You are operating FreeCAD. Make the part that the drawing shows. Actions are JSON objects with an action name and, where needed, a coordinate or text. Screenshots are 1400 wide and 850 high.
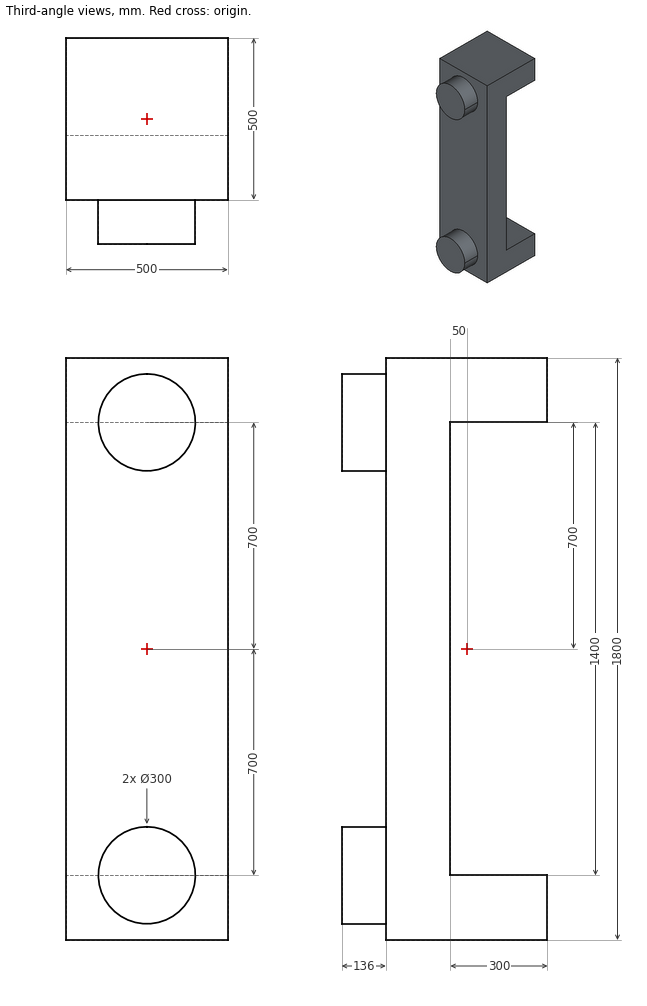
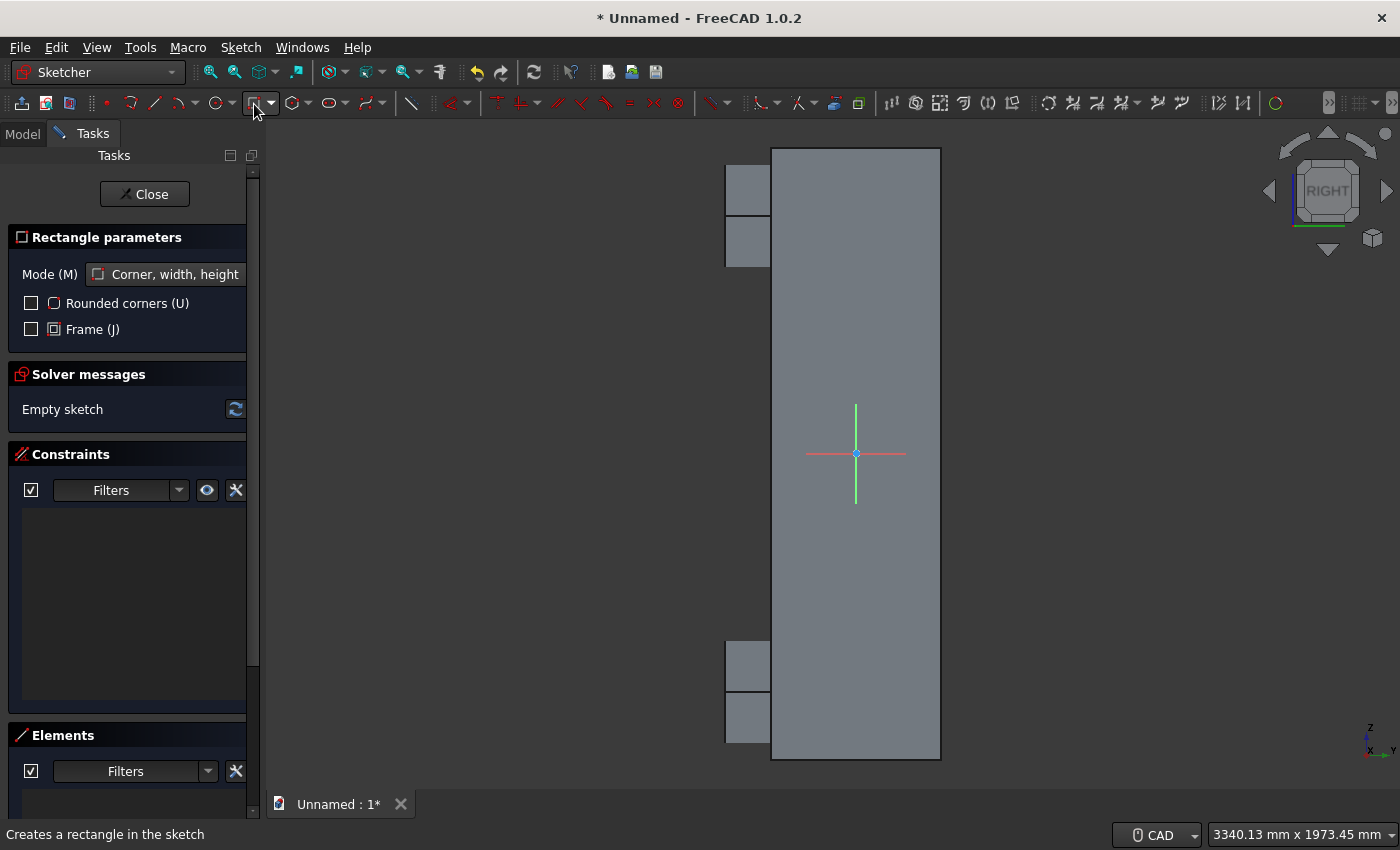
{"action": "left_click", "coordinate": [839, 216]}
{"action": "left_click", "coordinate": [941, 692]}
{"action": "key", "text": "Escape"}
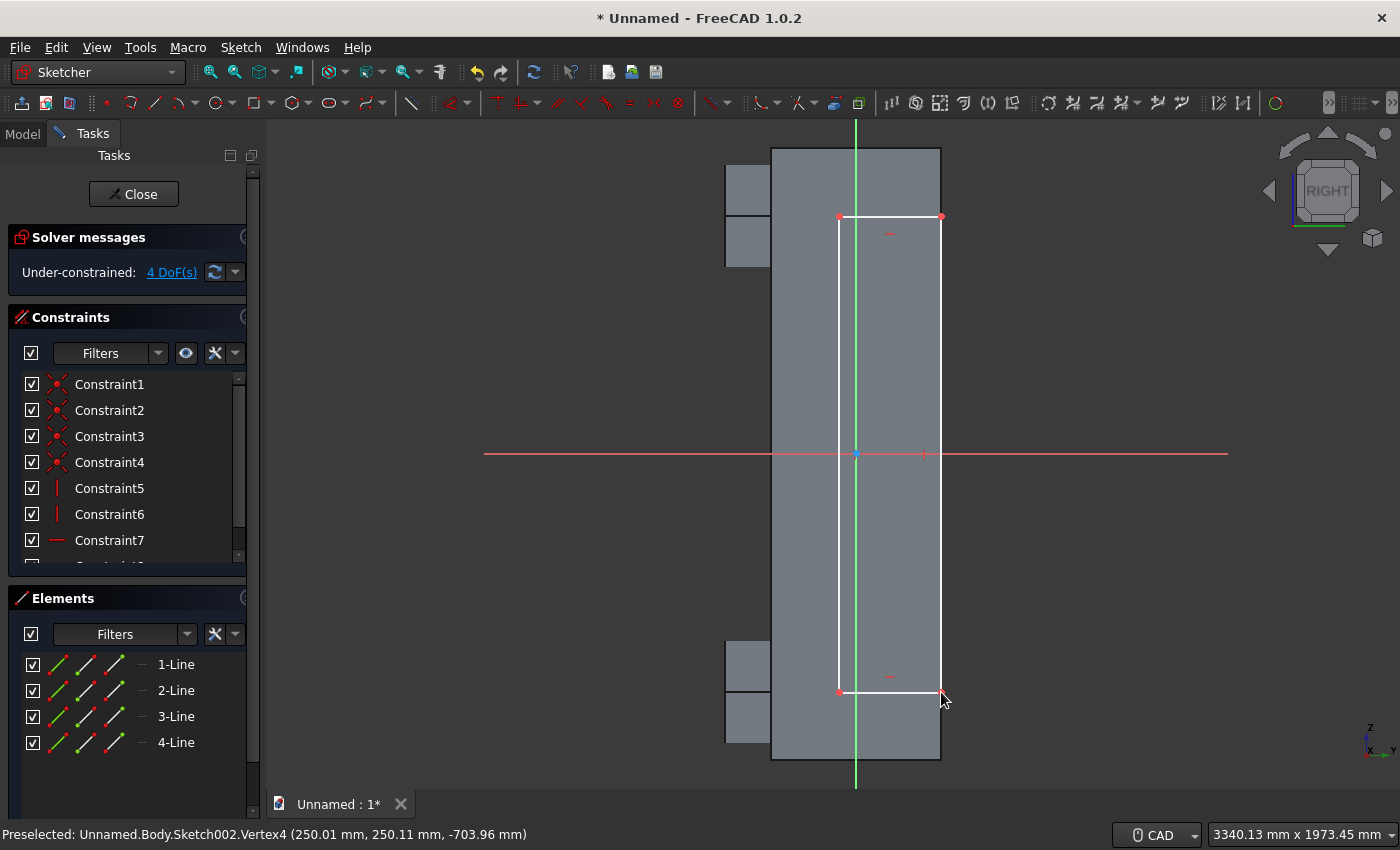
{"action": "left_click", "coordinate": [450, 104]}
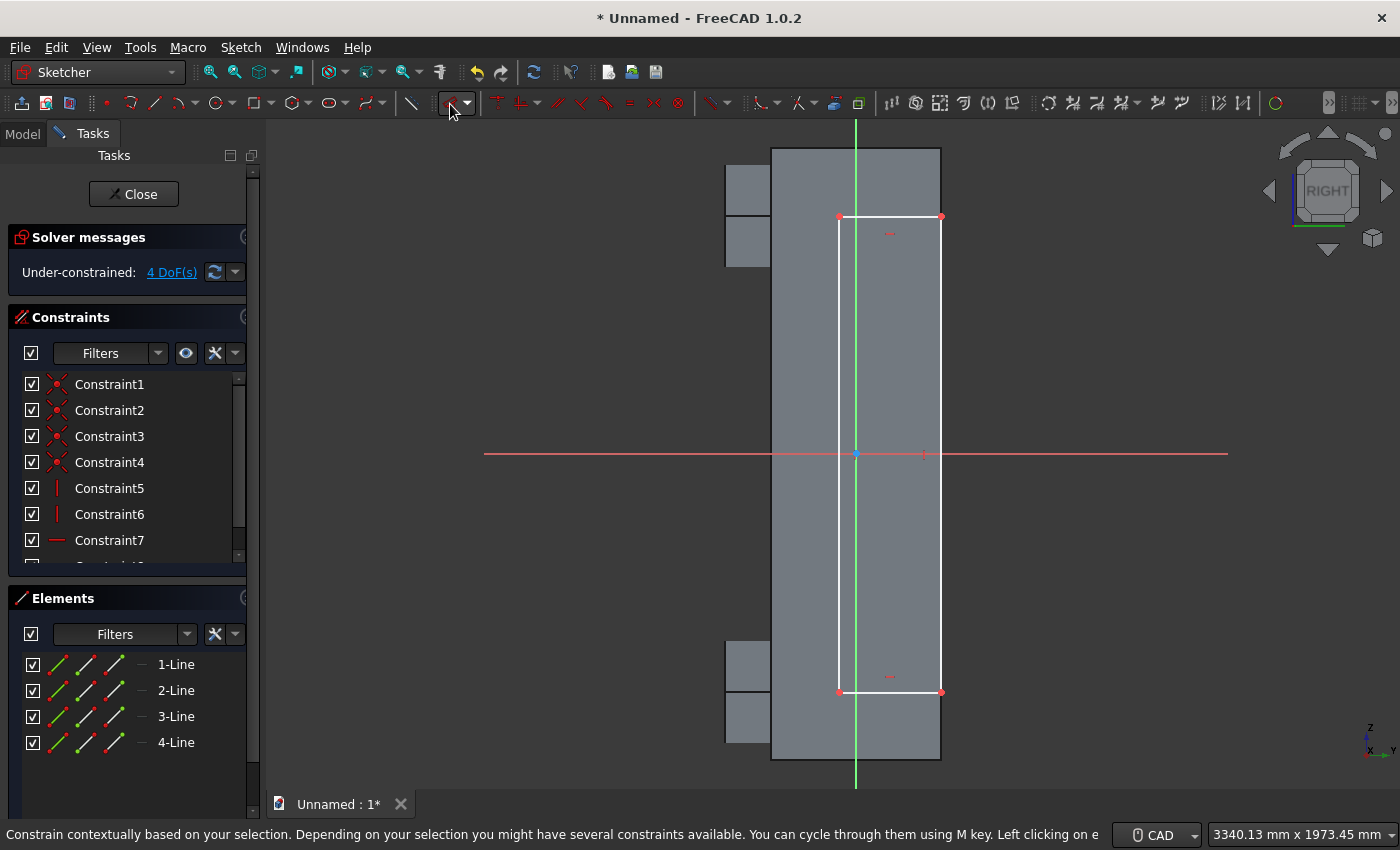
{"action": "left_click", "coordinate": [870, 693]}
{"action": "left_click", "coordinate": [890, 727]}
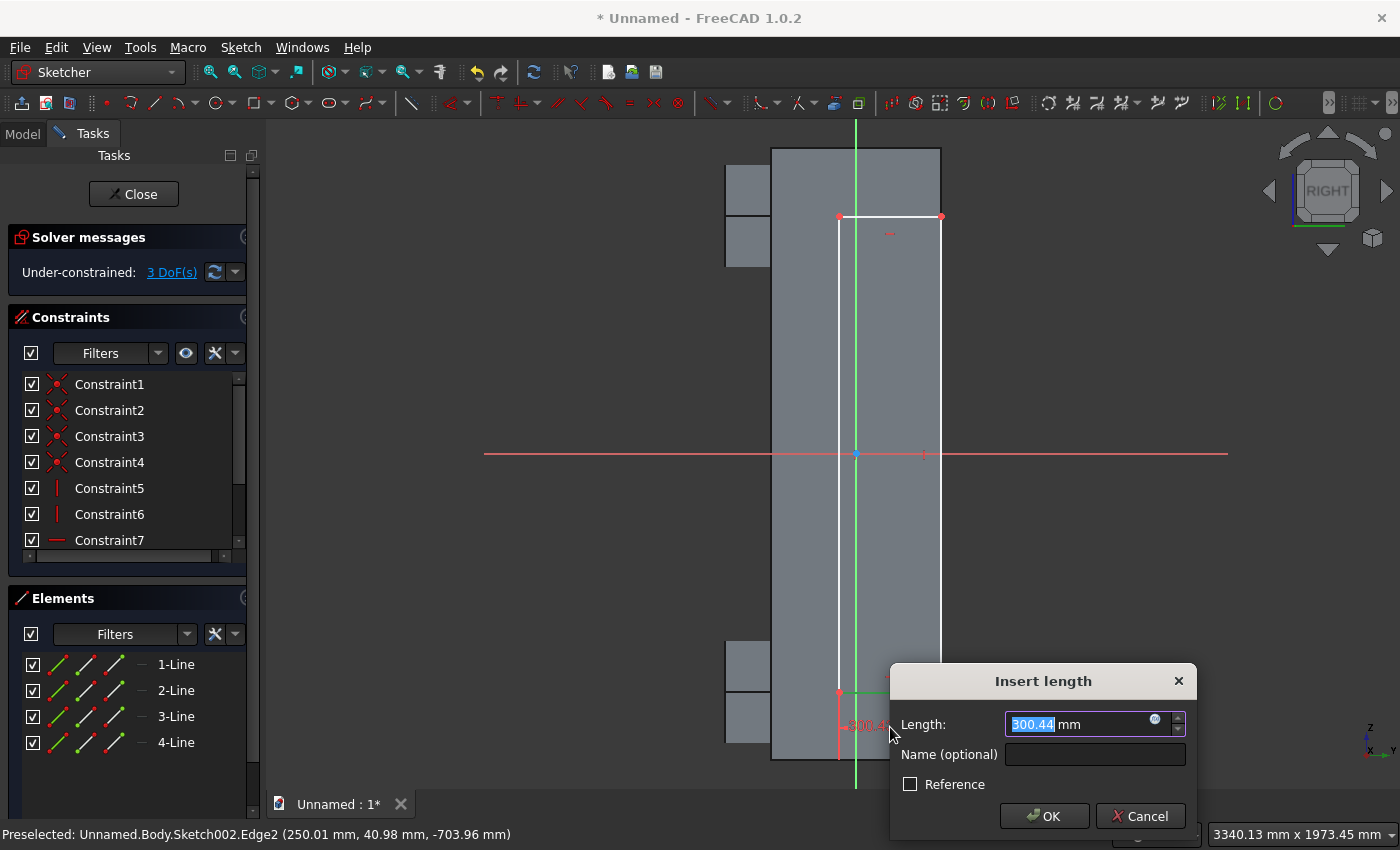
{"action": "type", "text": "300"}
{"action": "key", "text": "Return"}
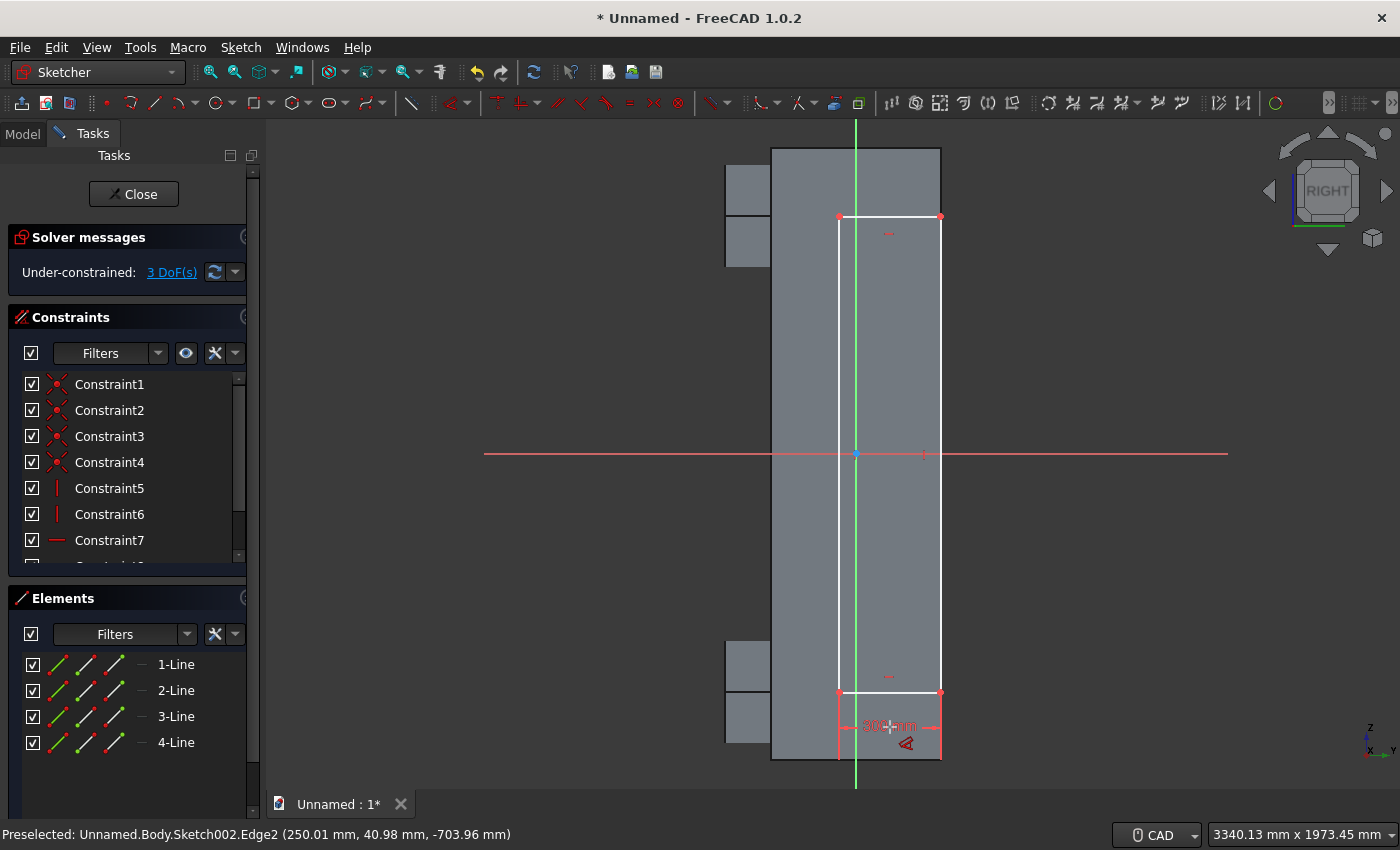
{"action": "scroll", "coordinate": [839, 217], "scroll_direction": "up", "scroll_amount": 5}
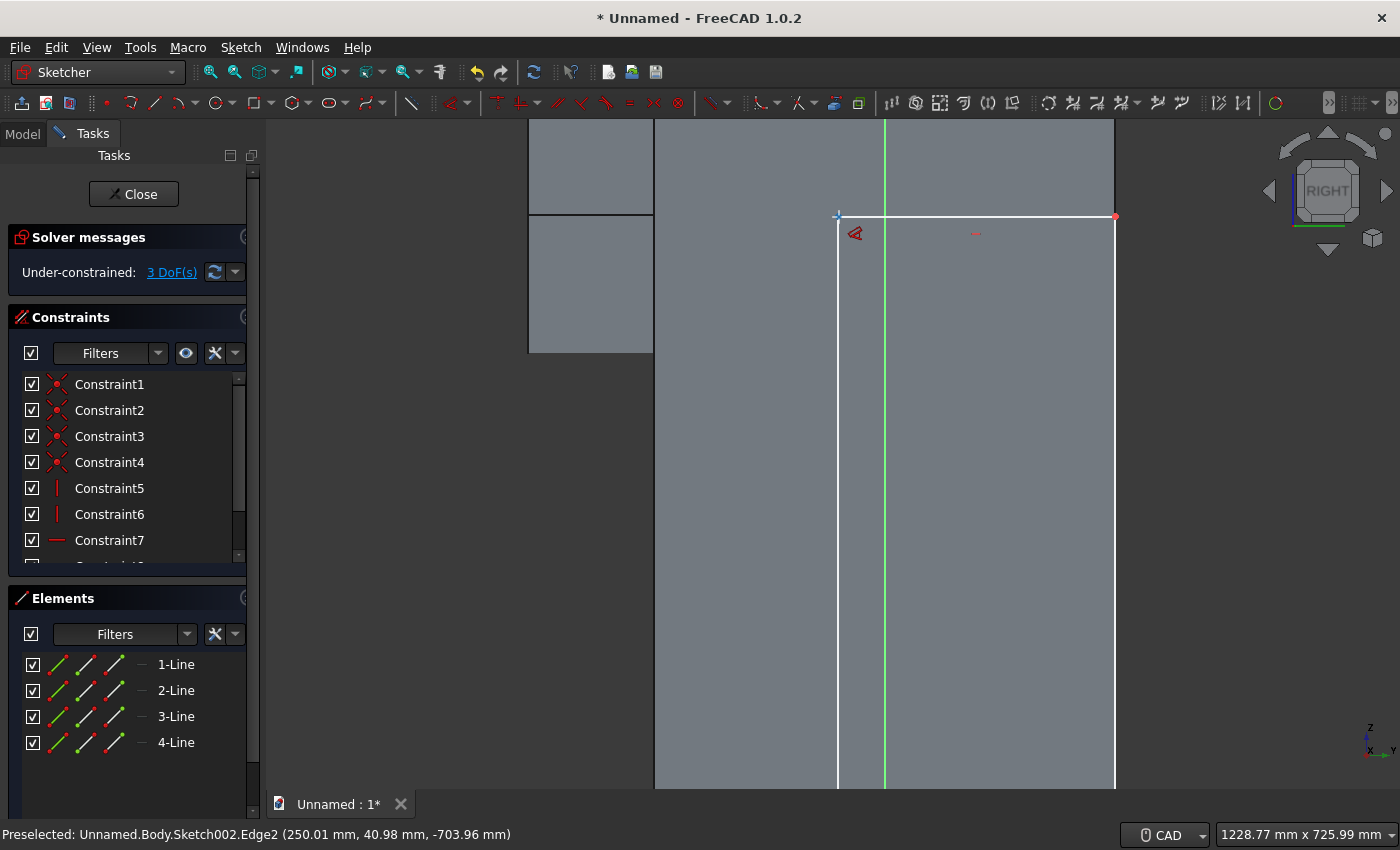
{"action": "left_click", "coordinate": [838, 217]}
{"action": "left_click", "coordinate": [861, 183]}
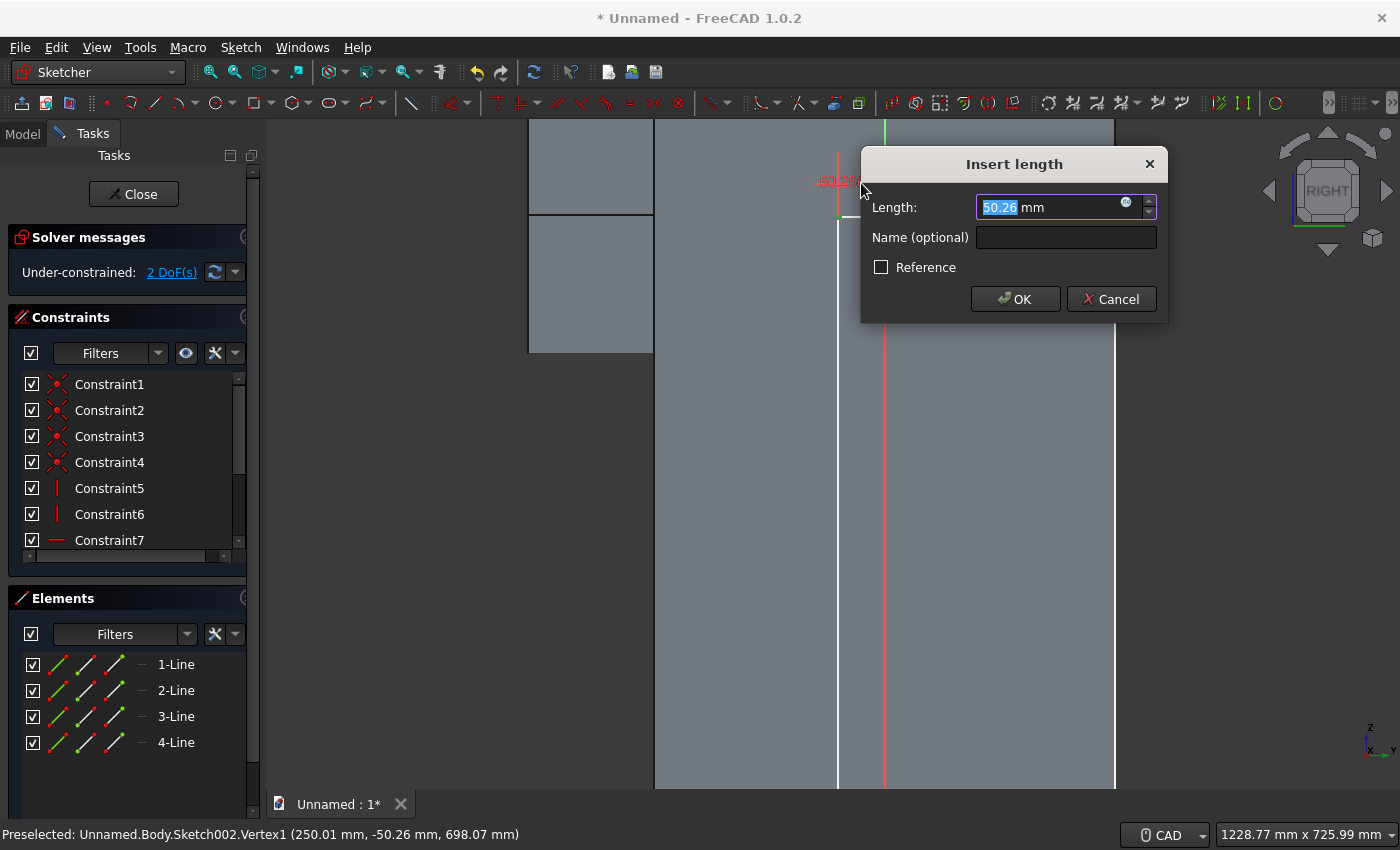
{"action": "type", "text": "50"}
{"action": "key", "text": "Return"}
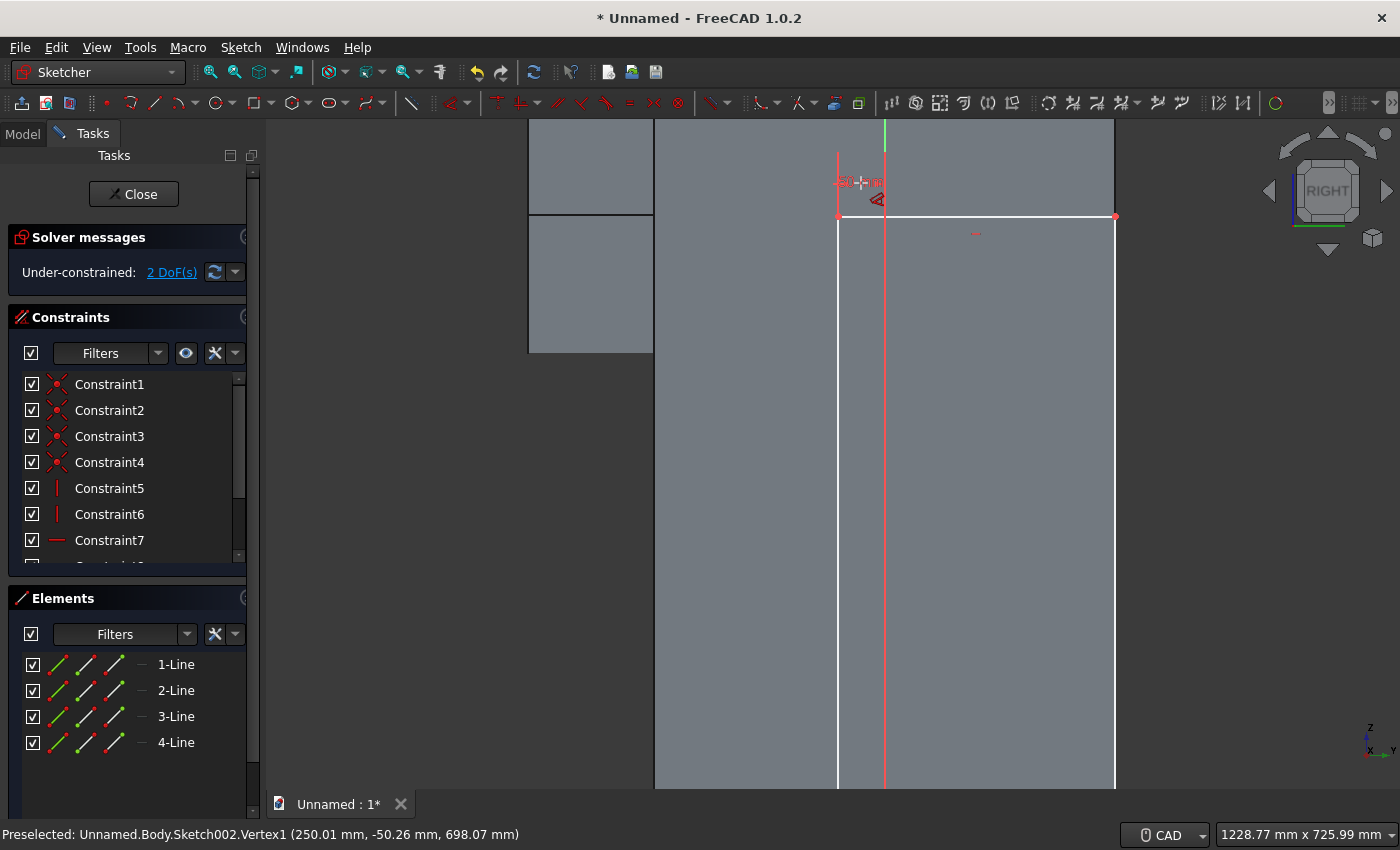
{"action": "left_click", "coordinate": [838, 605]}
{"action": "left_click", "coordinate": [804, 489]}